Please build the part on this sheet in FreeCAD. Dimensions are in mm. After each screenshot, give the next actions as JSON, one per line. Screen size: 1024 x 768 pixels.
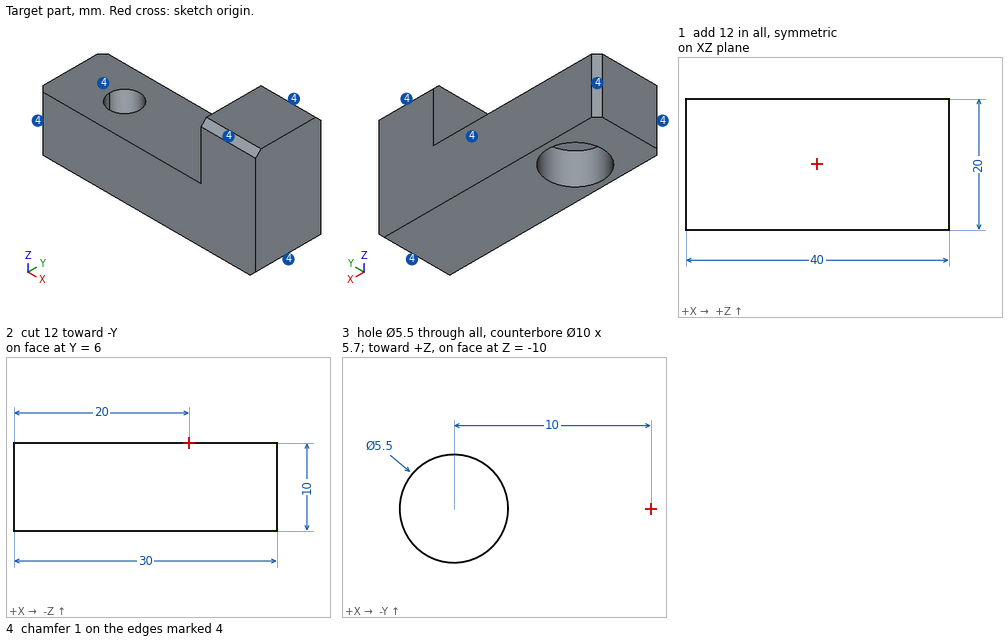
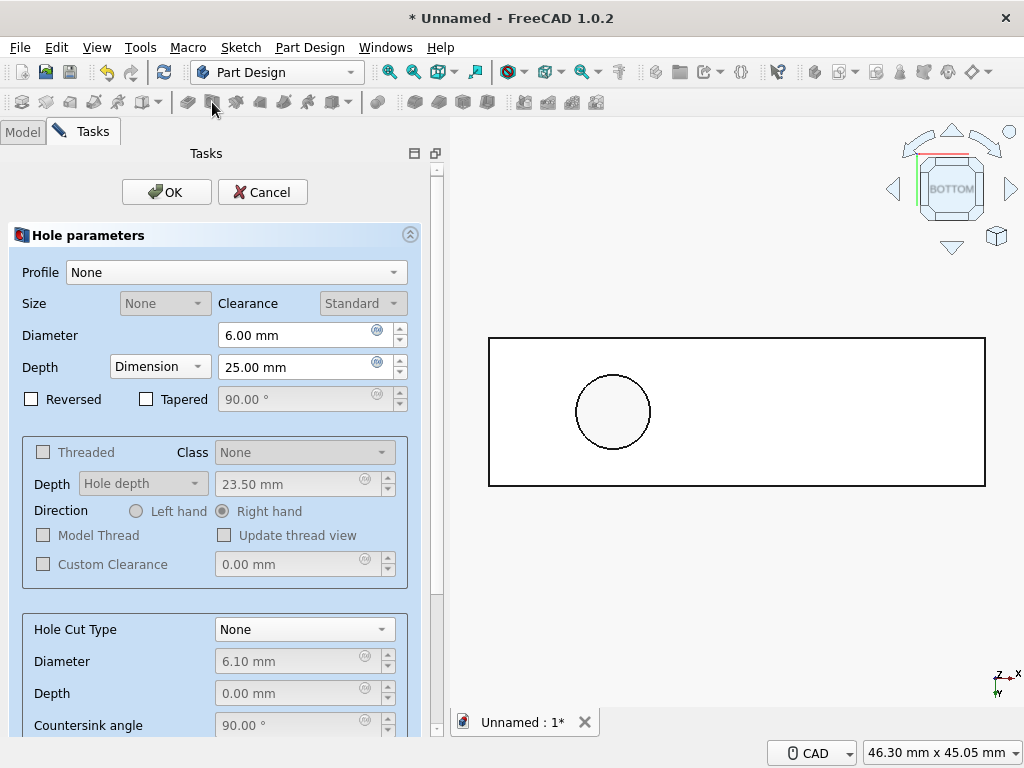
{"action": "triple_click", "coordinate": [305, 335]}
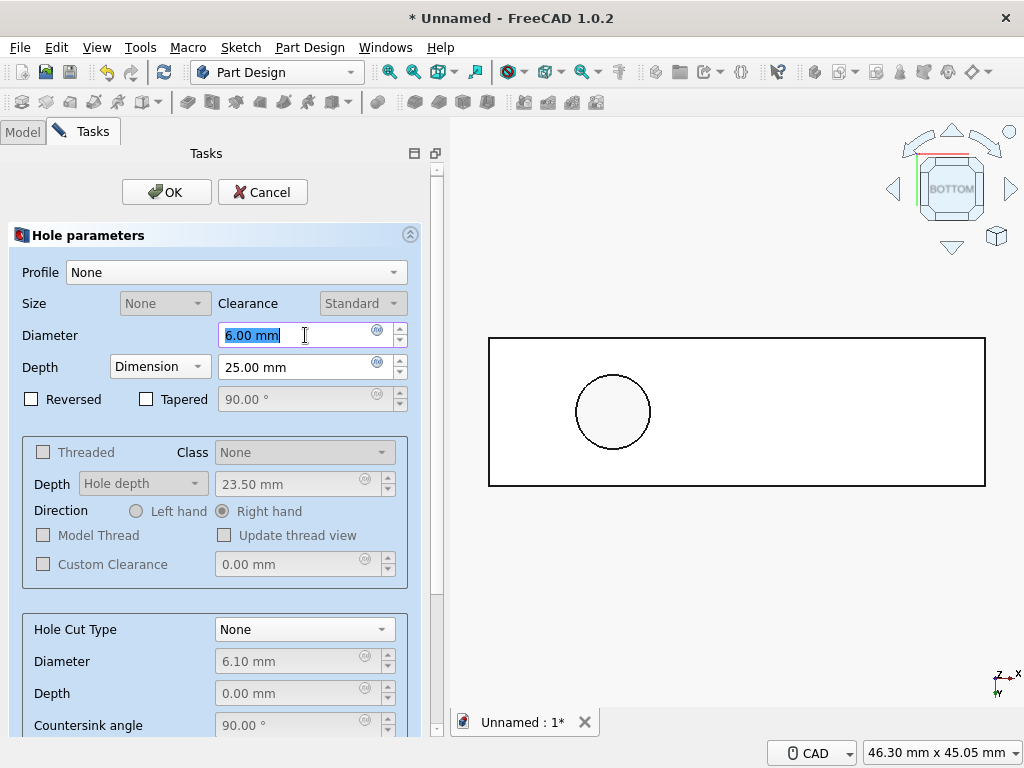
{"action": "type", "text": "5.5"}
{"action": "key", "text": "Tab"}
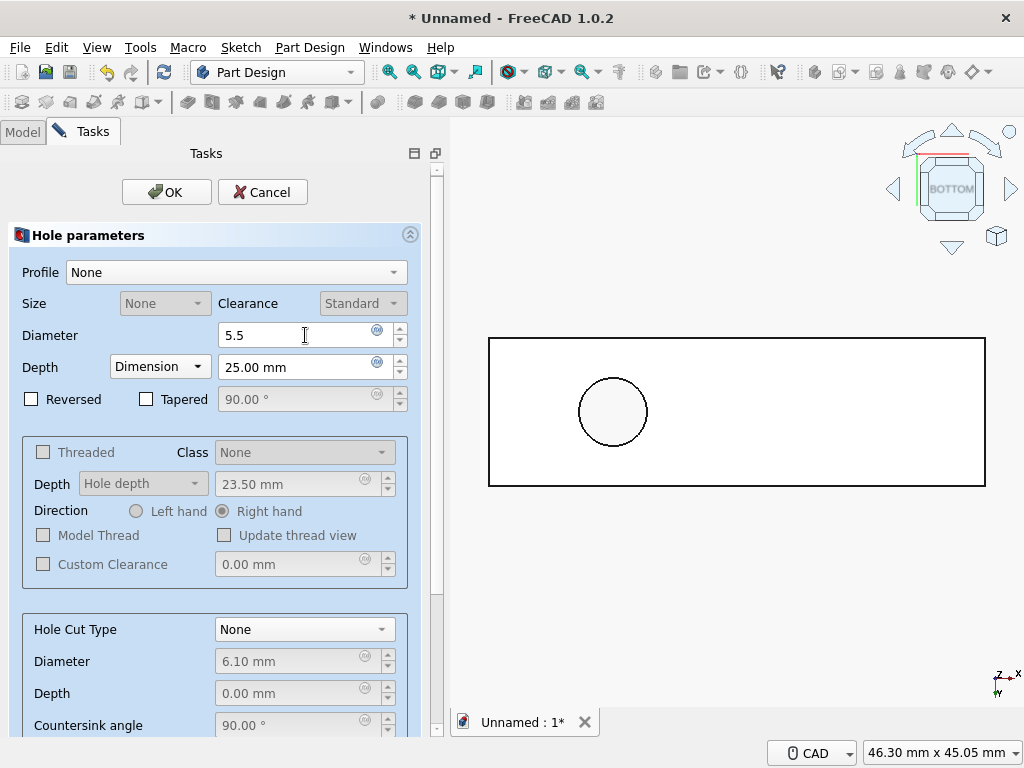
{"action": "left_click", "coordinate": [161, 366]}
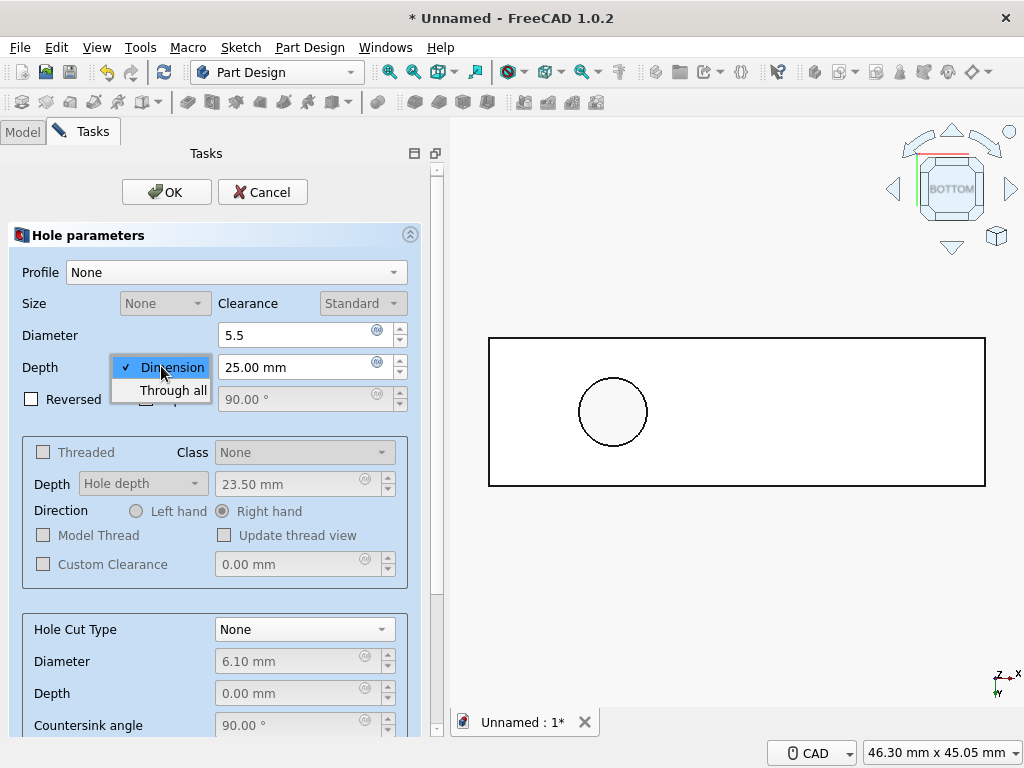
{"action": "left_click", "coordinate": [160, 390]}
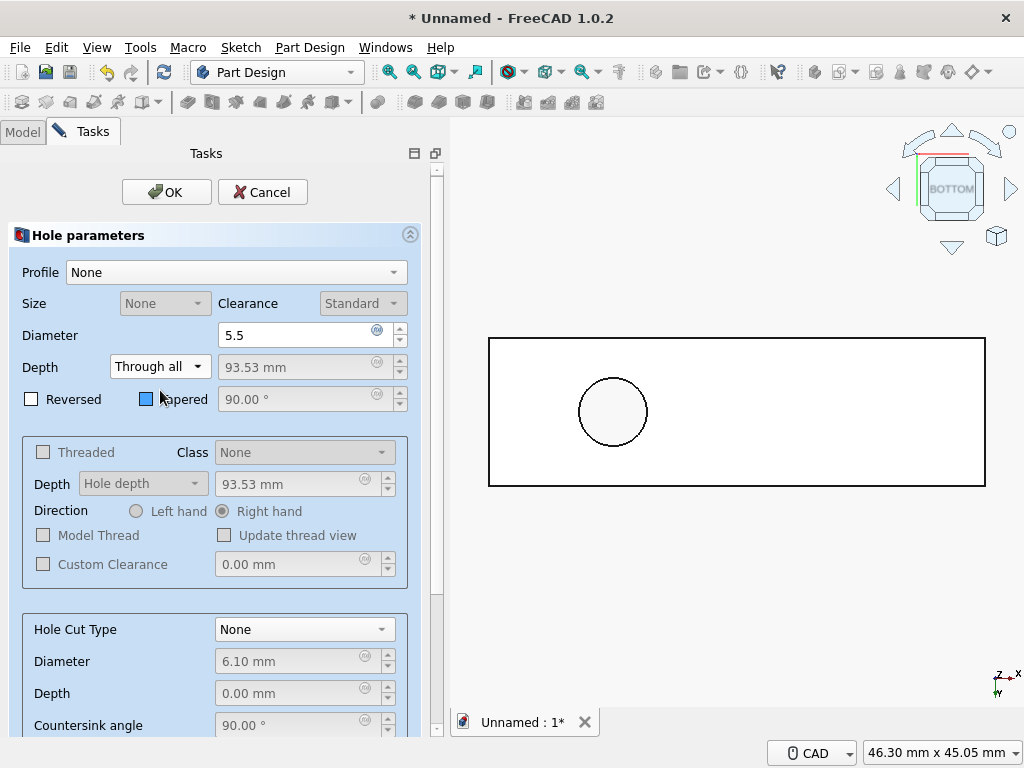
{"action": "left_click", "coordinate": [306, 630]}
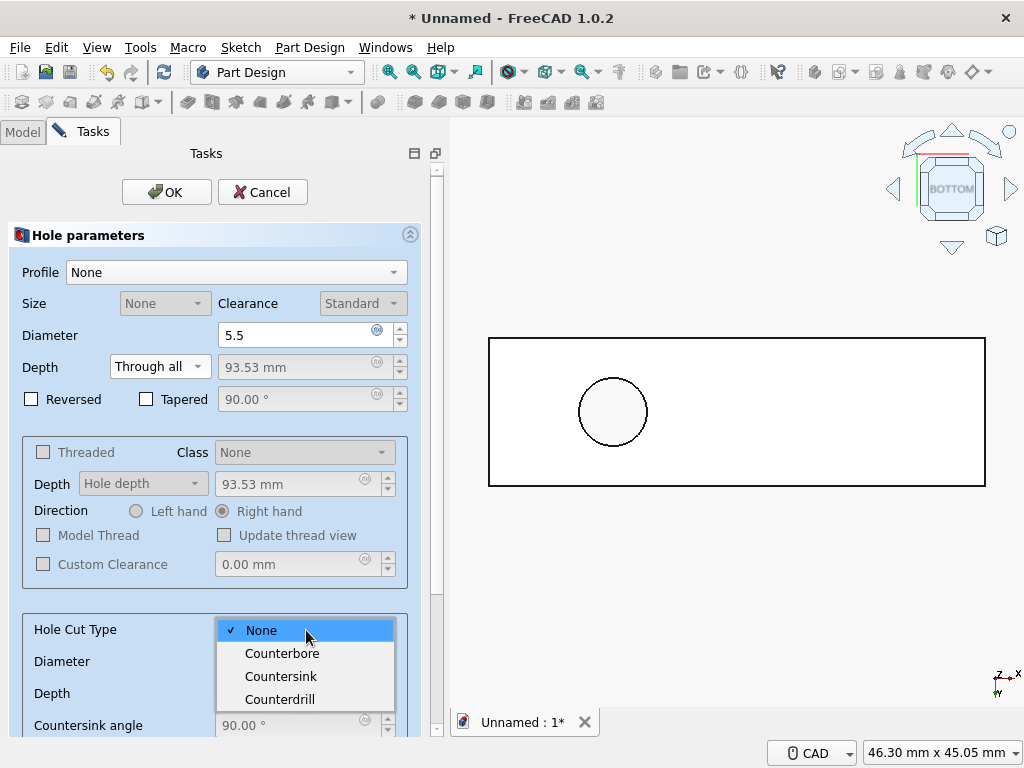
{"action": "left_click", "coordinate": [304, 654]}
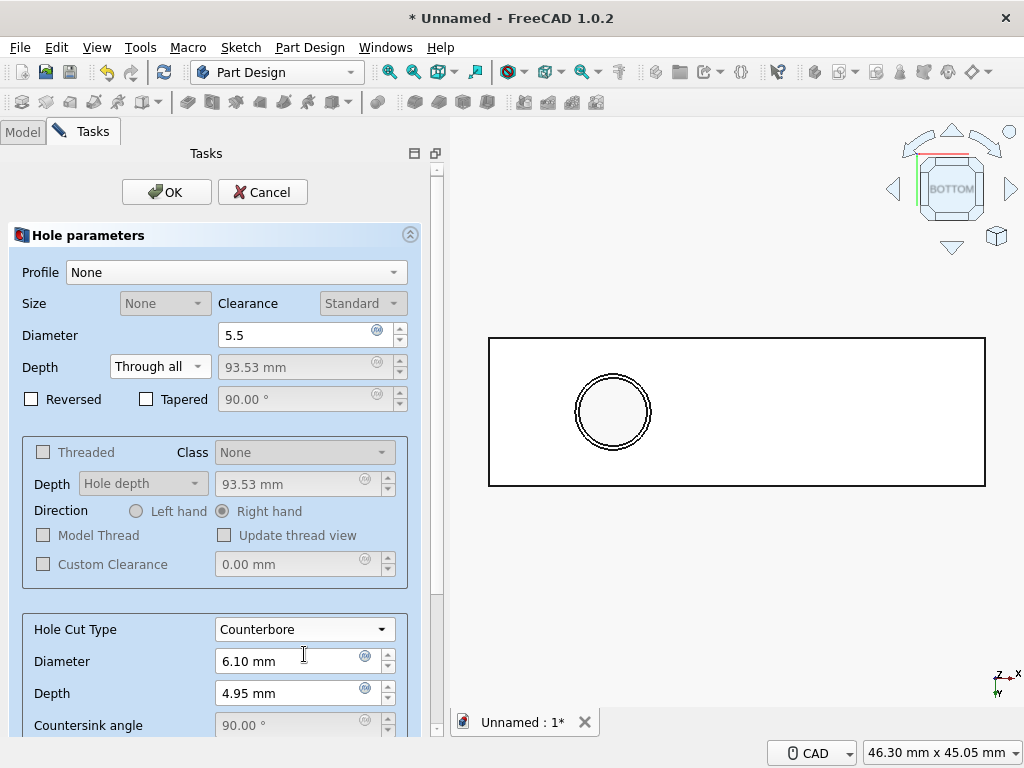
{"action": "triple_click", "coordinate": [298, 661]}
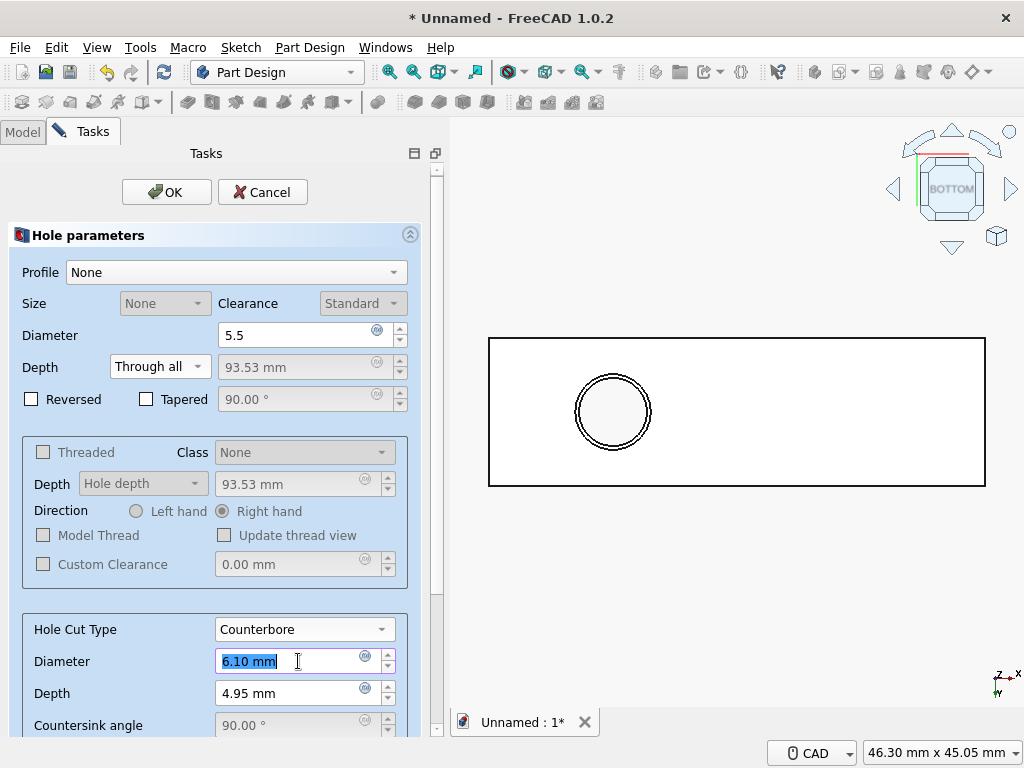
{"action": "type", "text": "10"}
{"action": "key", "text": "Tab"}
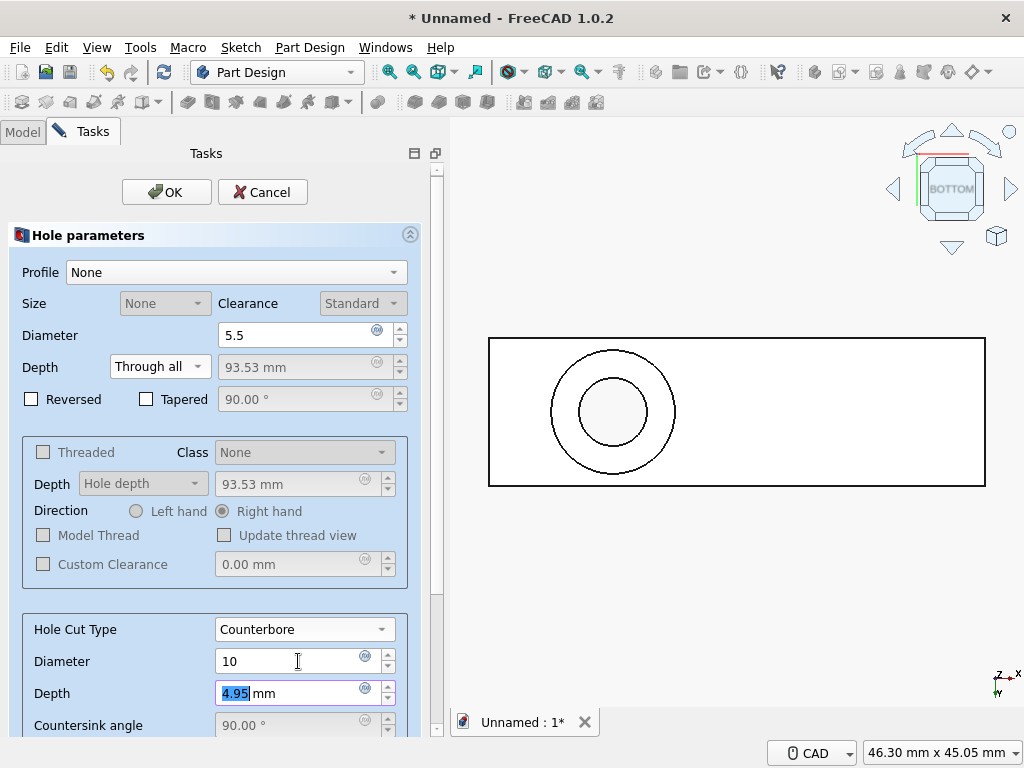
{"action": "type", "text": "5.7"}
{"action": "key", "text": "Tab"}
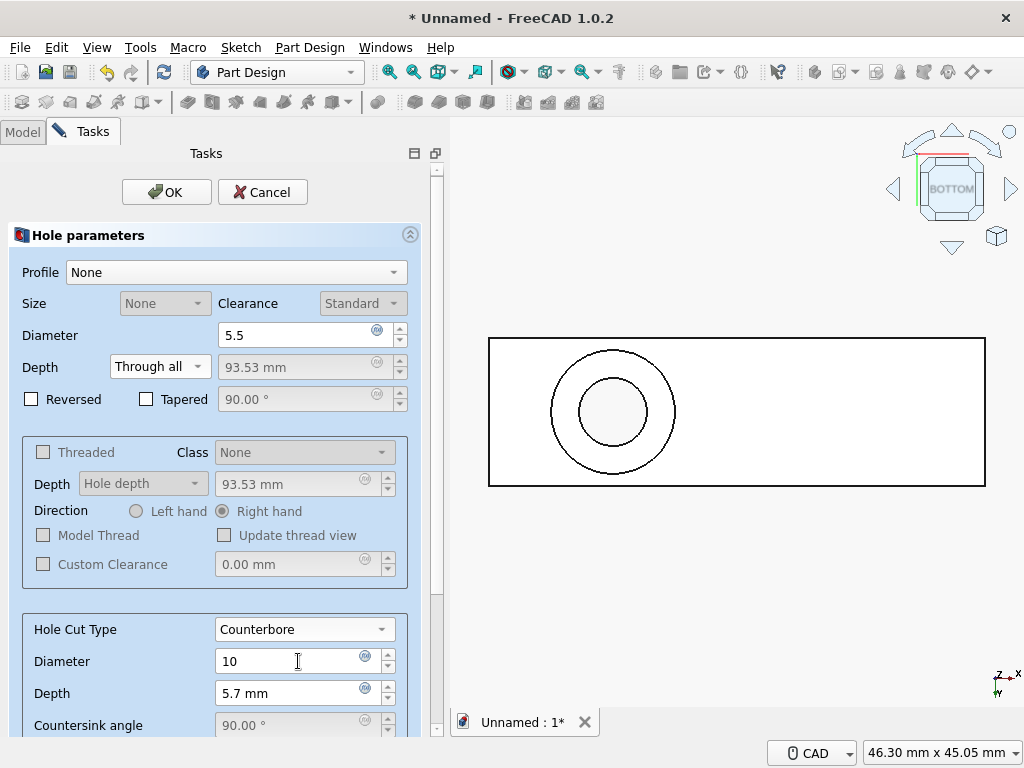
{"action": "left_click", "coordinate": [167, 192]}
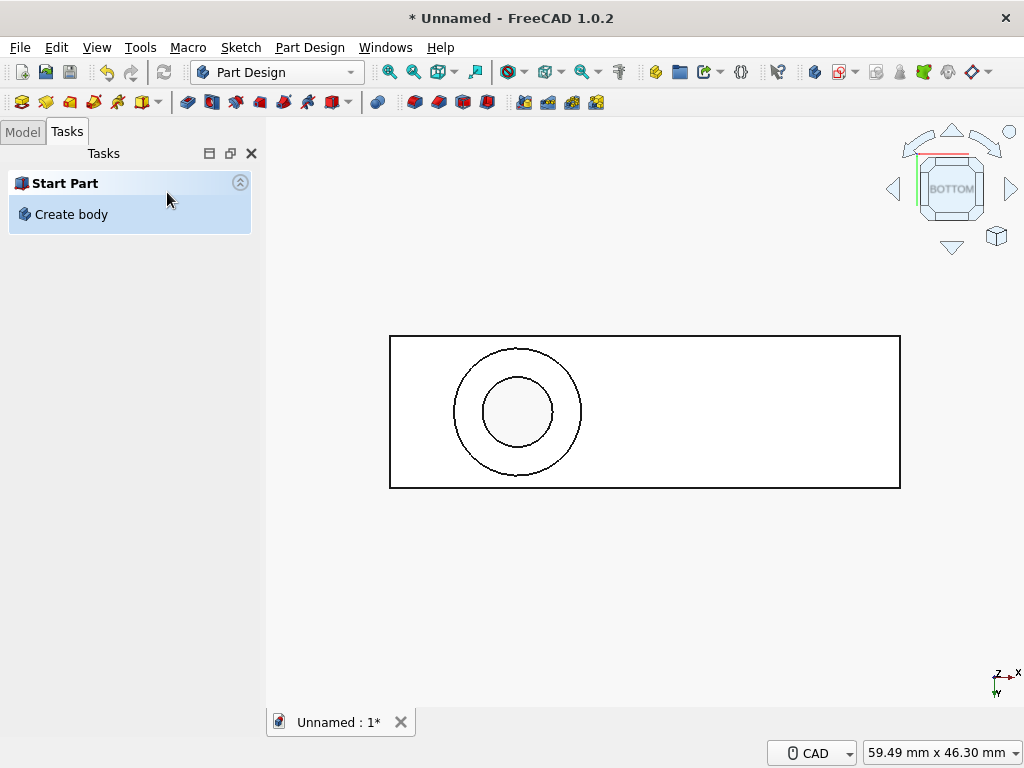
{"action": "left_click", "coordinate": [900, 411]}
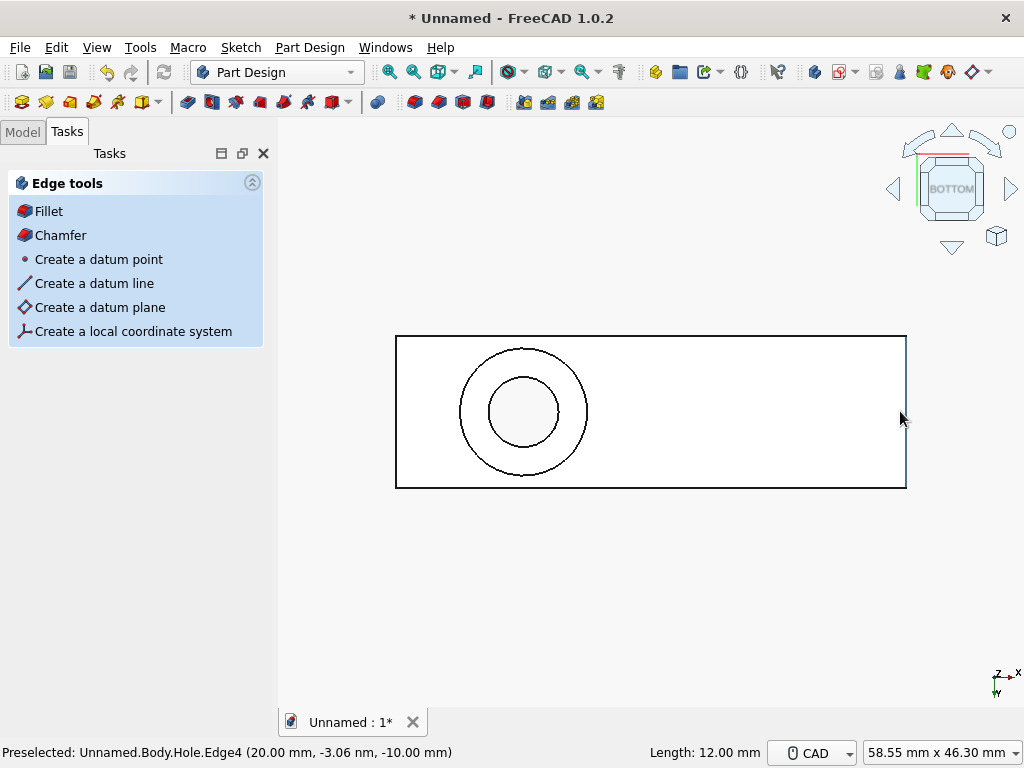
{"action": "key", "text": "0"}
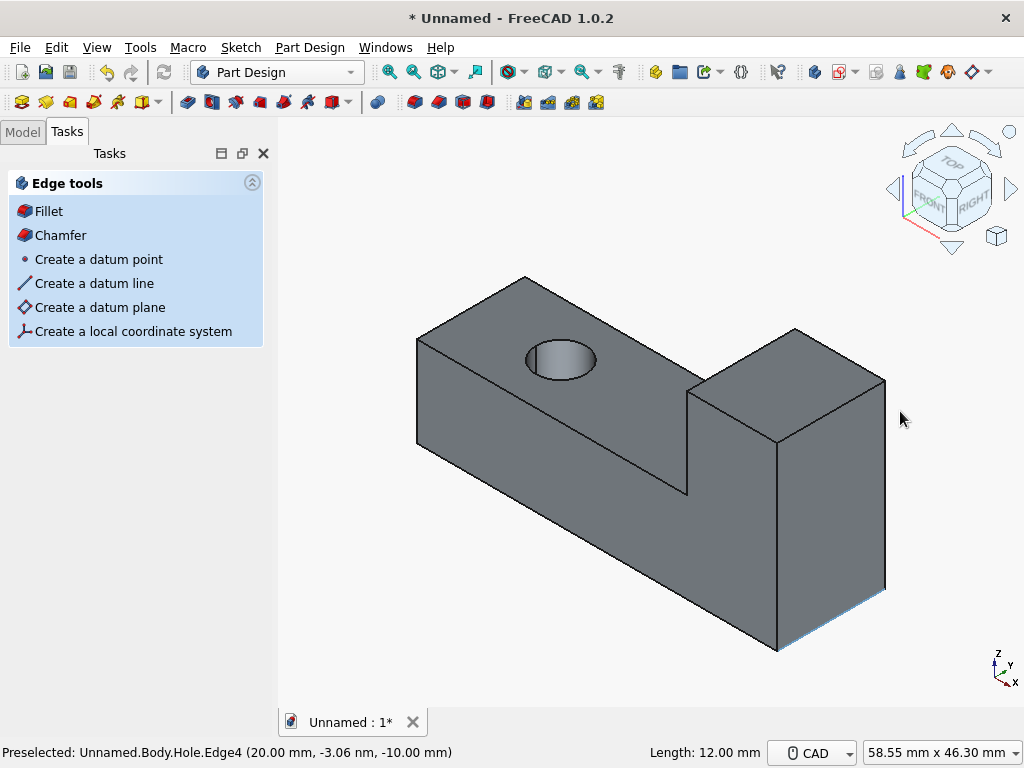
{"action": "left_click", "coordinate": [732, 416], "text": "ctrl"}